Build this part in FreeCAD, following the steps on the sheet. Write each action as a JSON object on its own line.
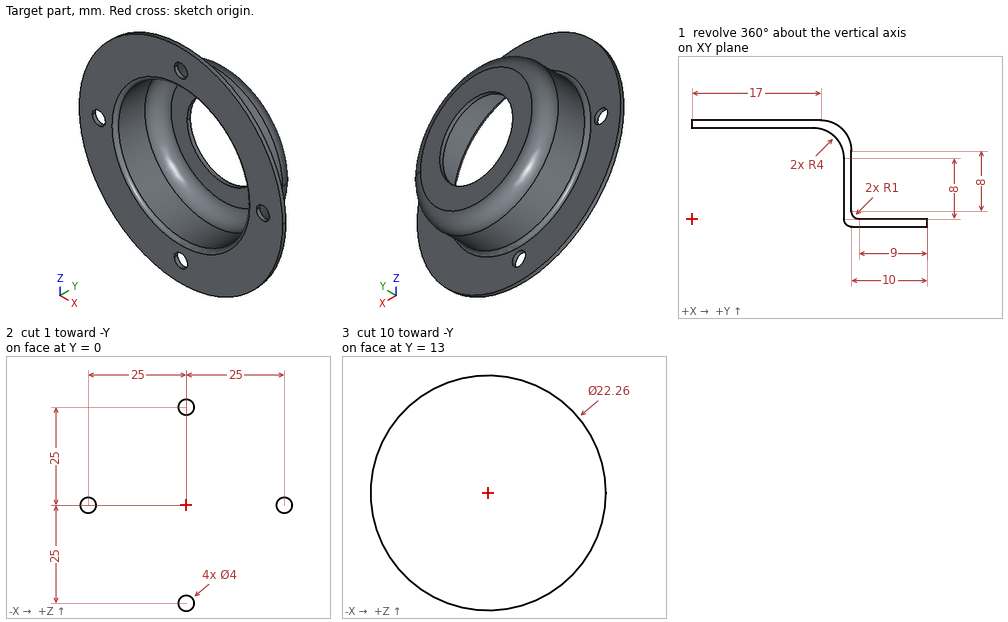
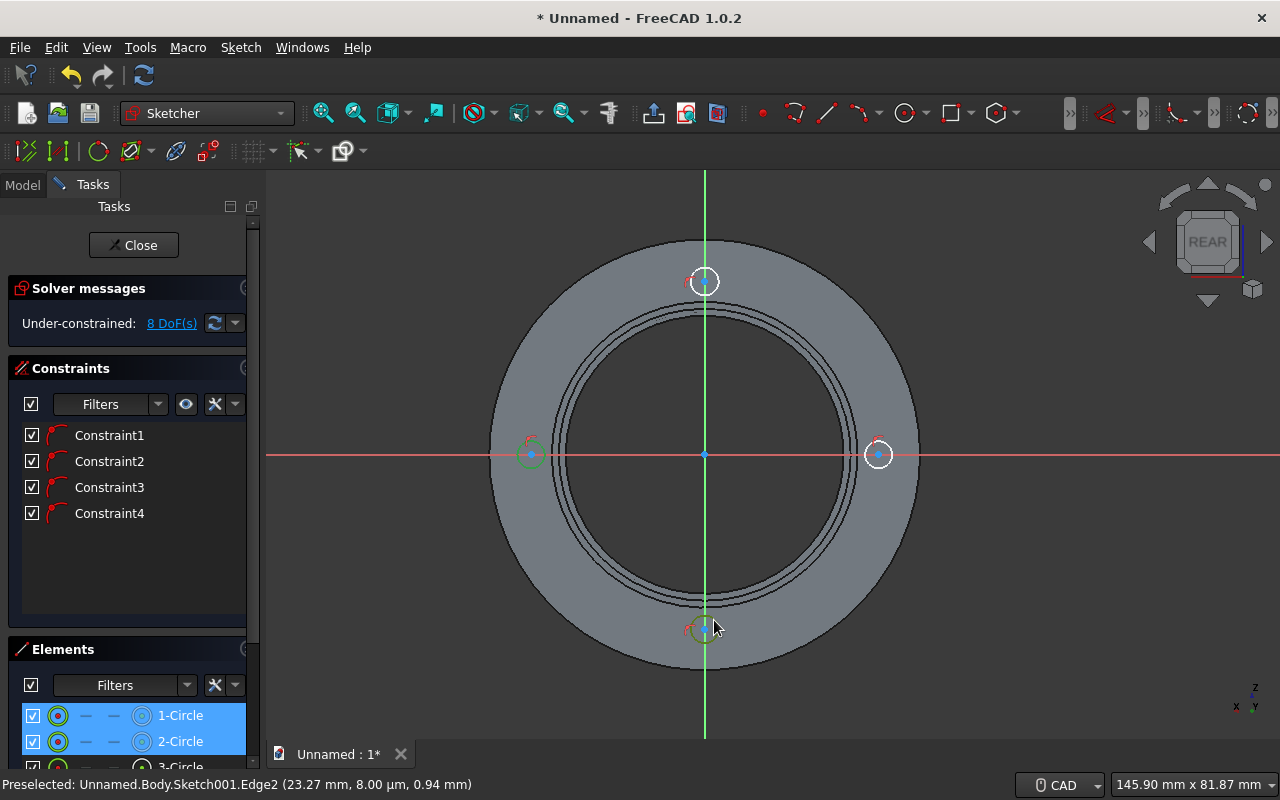
{"action": "scroll", "coordinate": [715, 272], "scroll_direction": "up", "scroll_amount": 2}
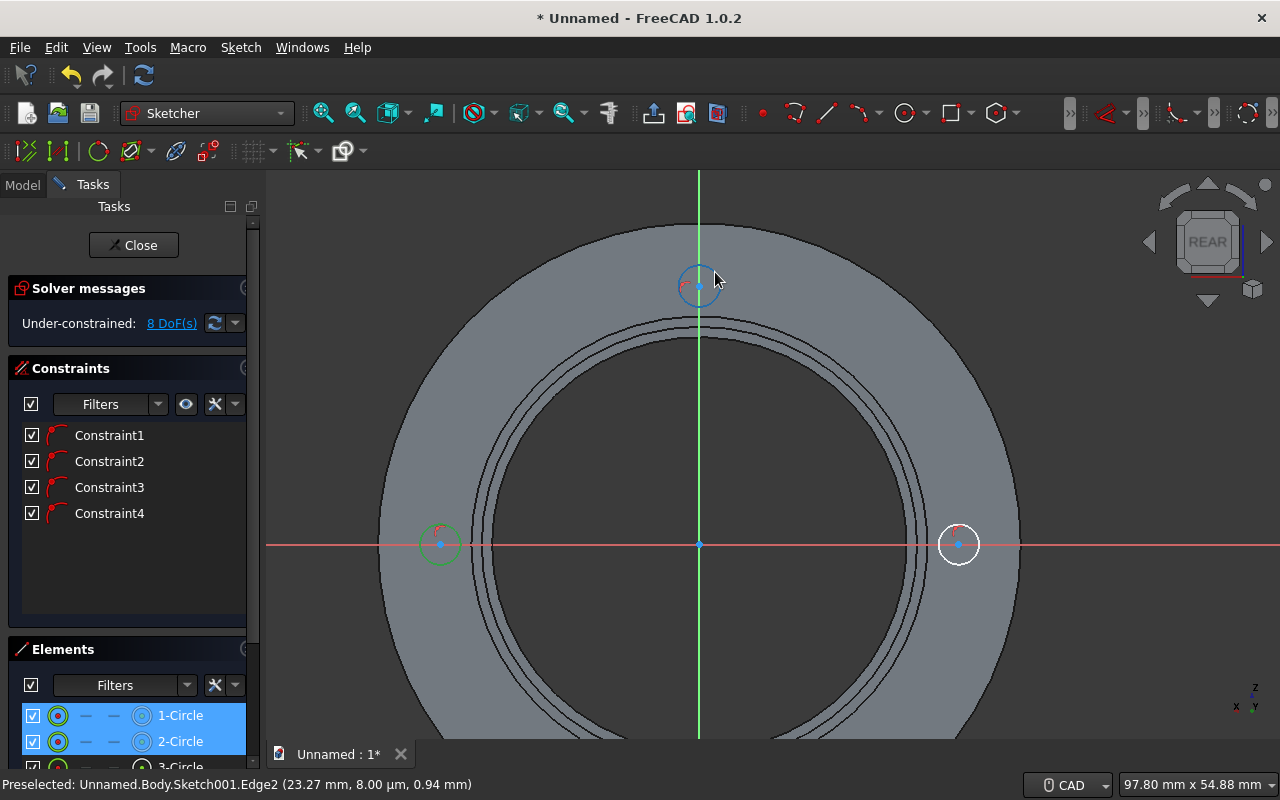
{"action": "left_click", "coordinate": [714, 271]}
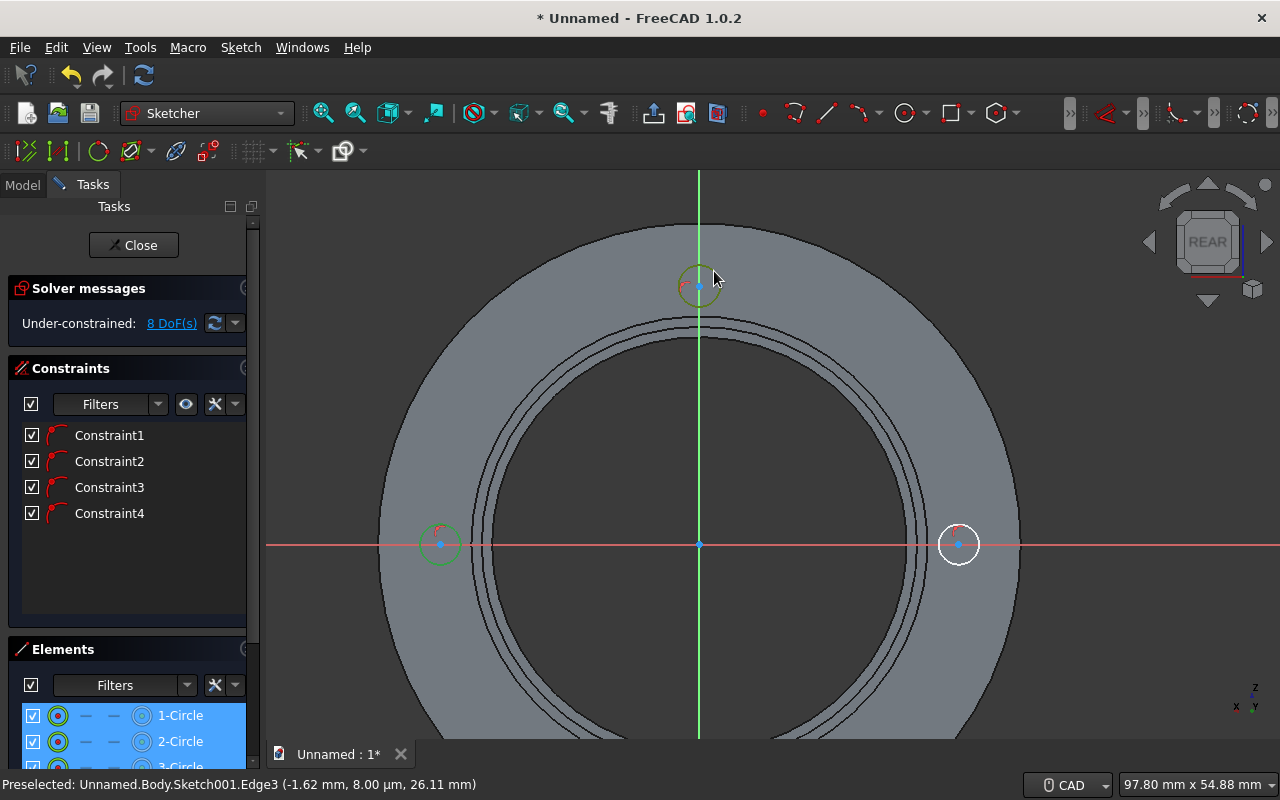
{"action": "left_click", "coordinate": [973, 530]}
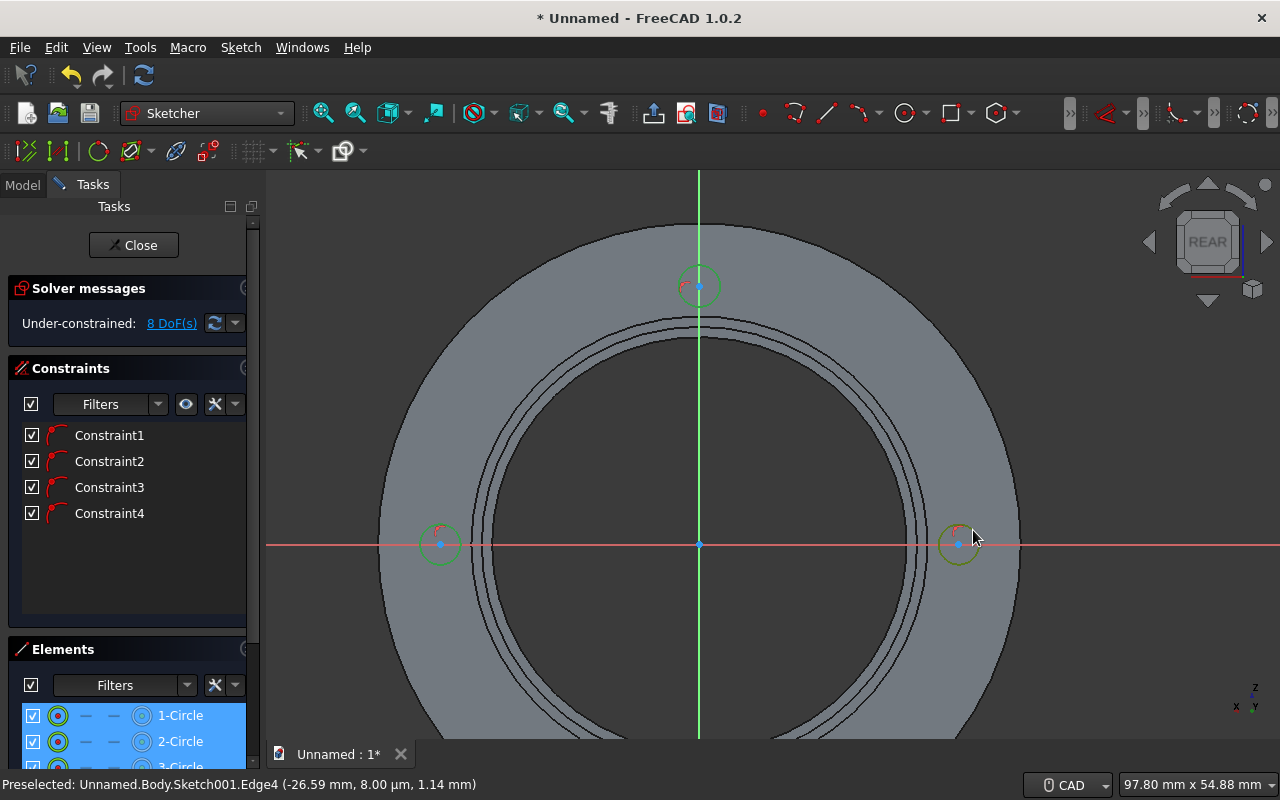
{"action": "key", "text": "e"}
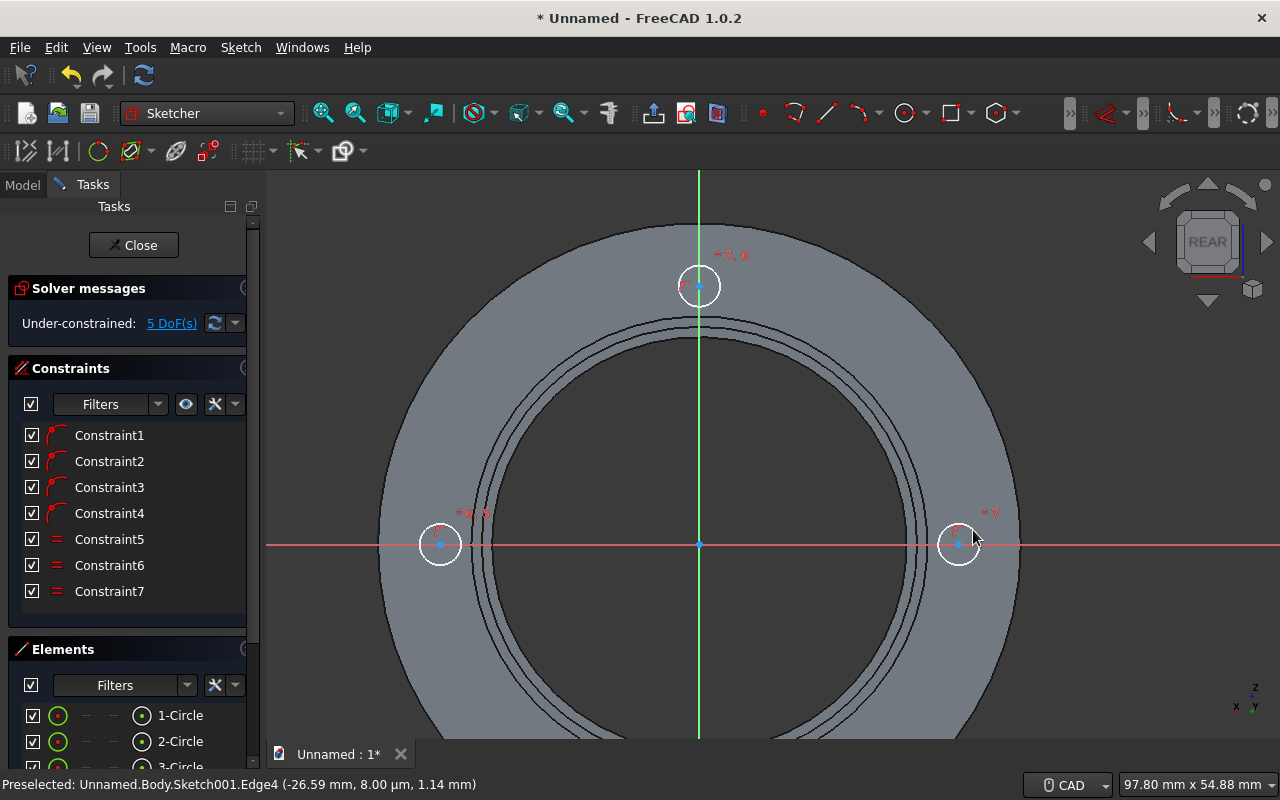
{"action": "left_click", "coordinate": [1106, 114]}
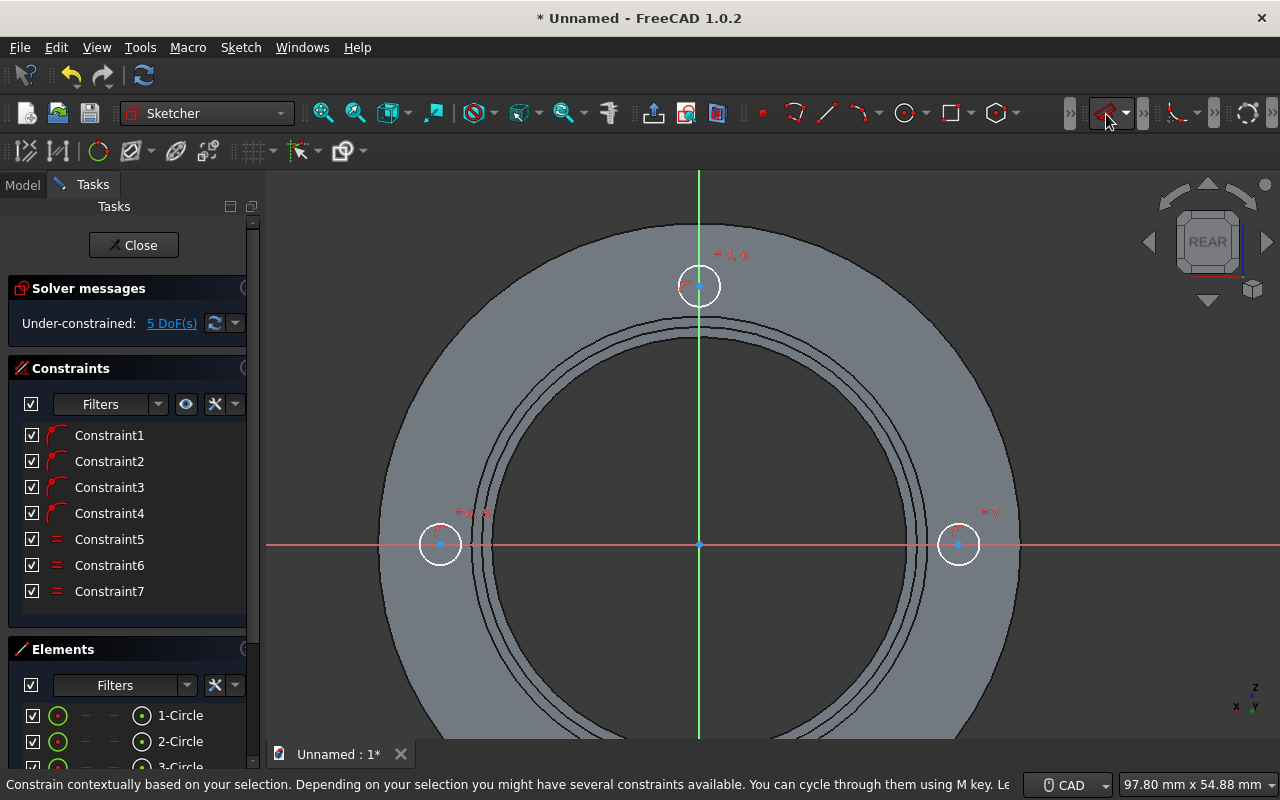
{"action": "scroll", "coordinate": [715, 271], "scroll_direction": "down", "scroll_amount": 2}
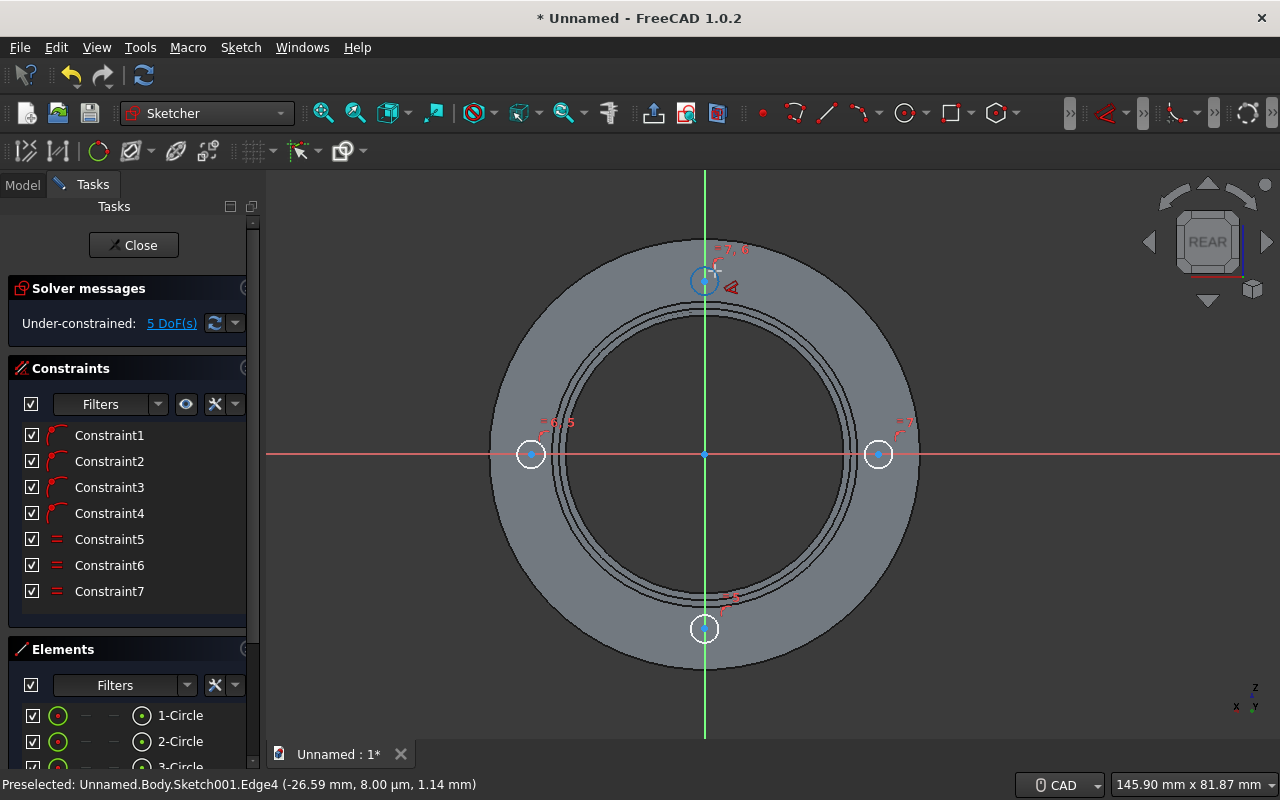
{"action": "scroll", "coordinate": [714, 619], "scroll_direction": "up", "scroll_amount": 2}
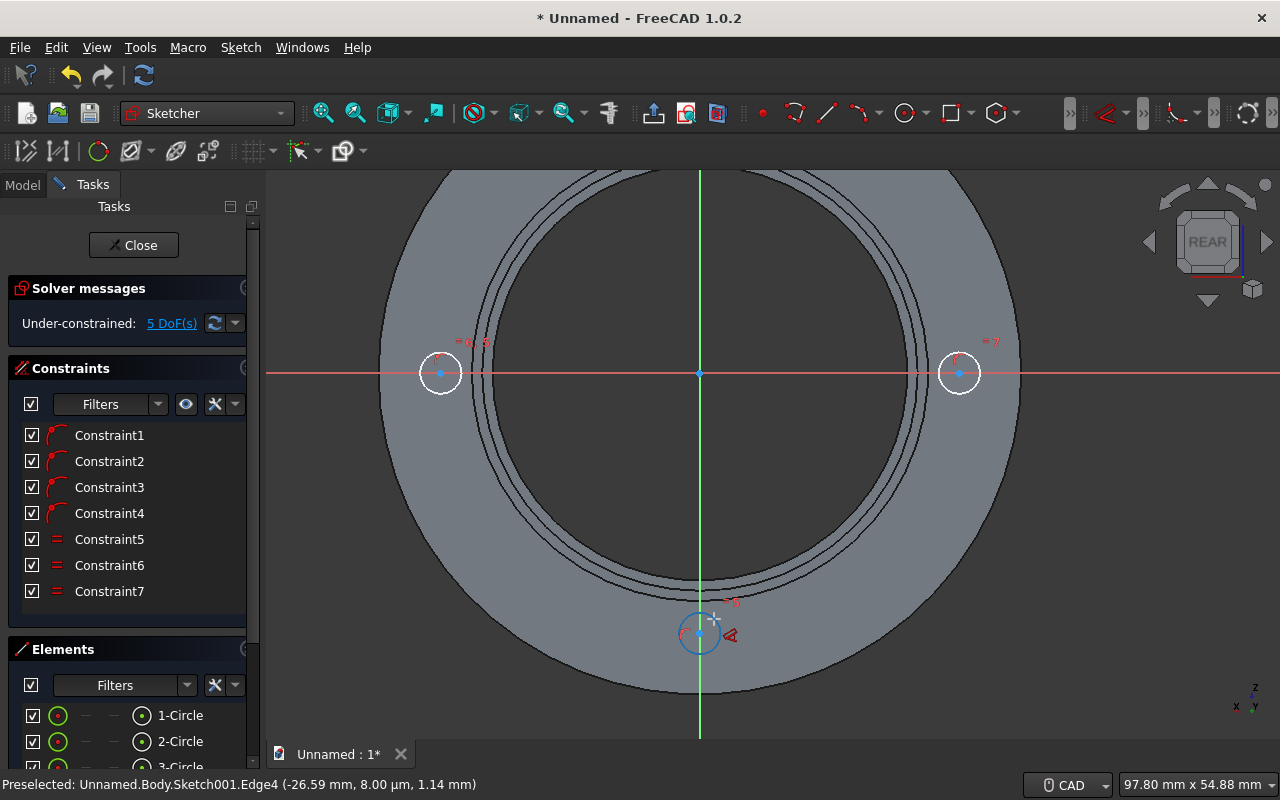
{"action": "left_click", "coordinate": [714, 619]}
{"action": "left_click", "coordinate": [736, 596]}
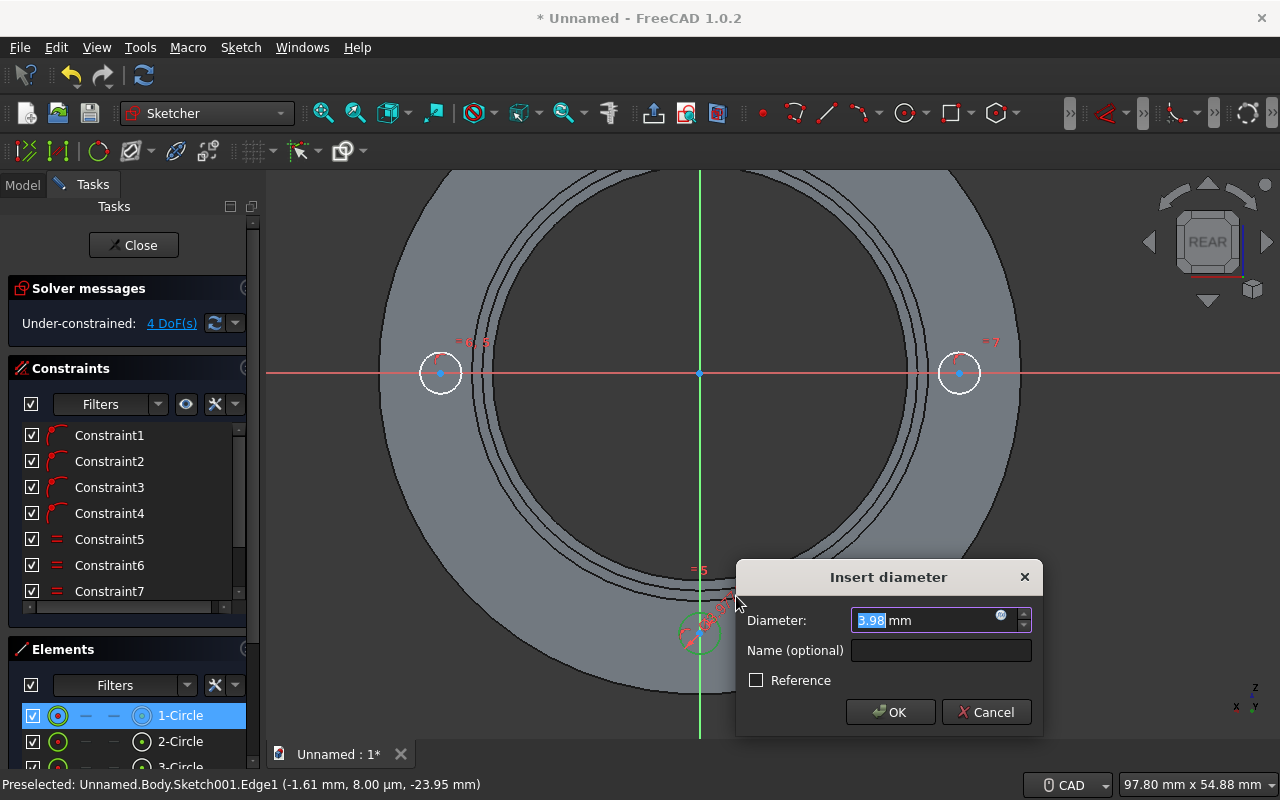
{"action": "type", "text": "4"}
{"action": "key", "text": "Return"}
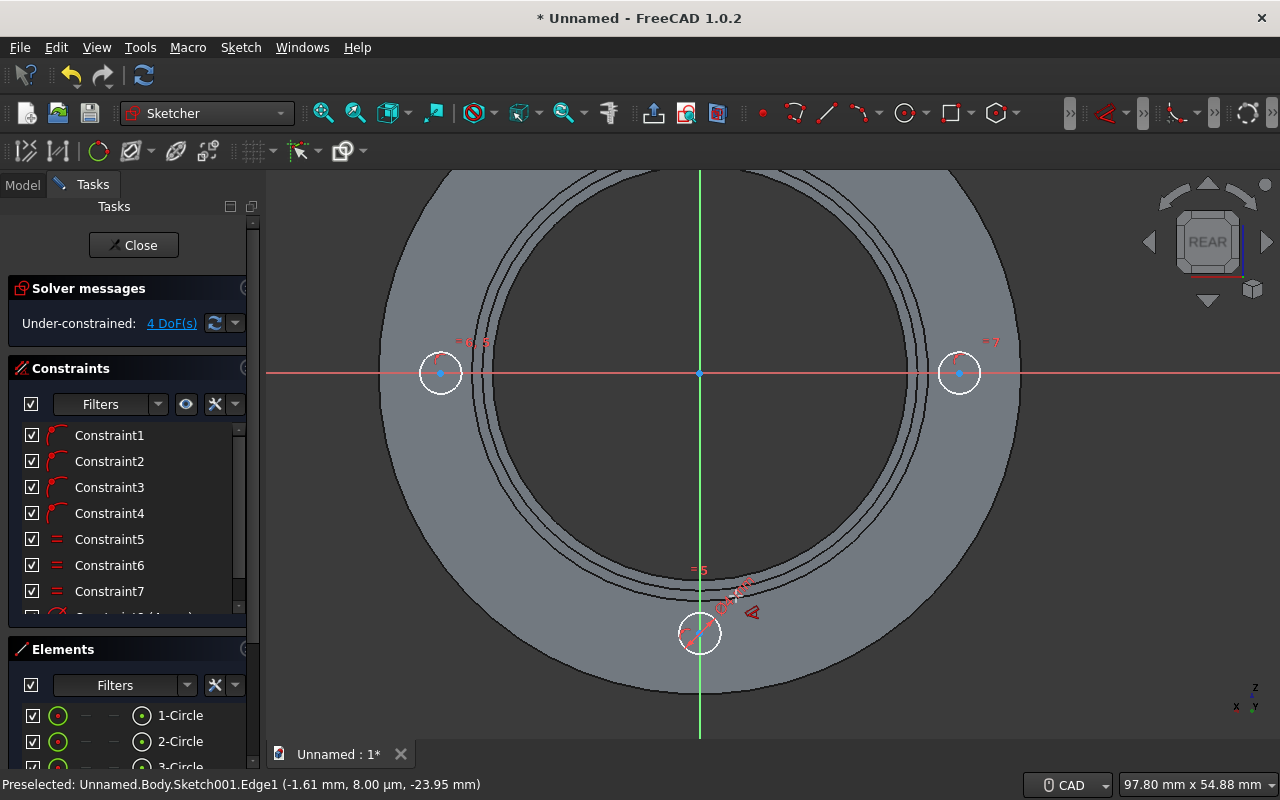
{"action": "left_click", "coordinate": [700, 633]}
{"action": "left_click", "coordinate": [734, 503]}